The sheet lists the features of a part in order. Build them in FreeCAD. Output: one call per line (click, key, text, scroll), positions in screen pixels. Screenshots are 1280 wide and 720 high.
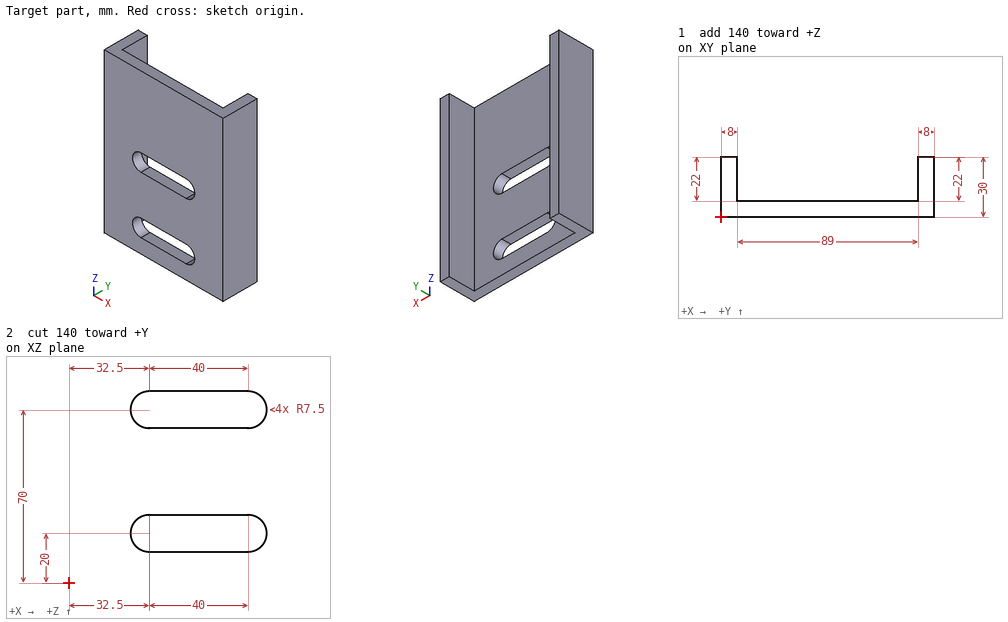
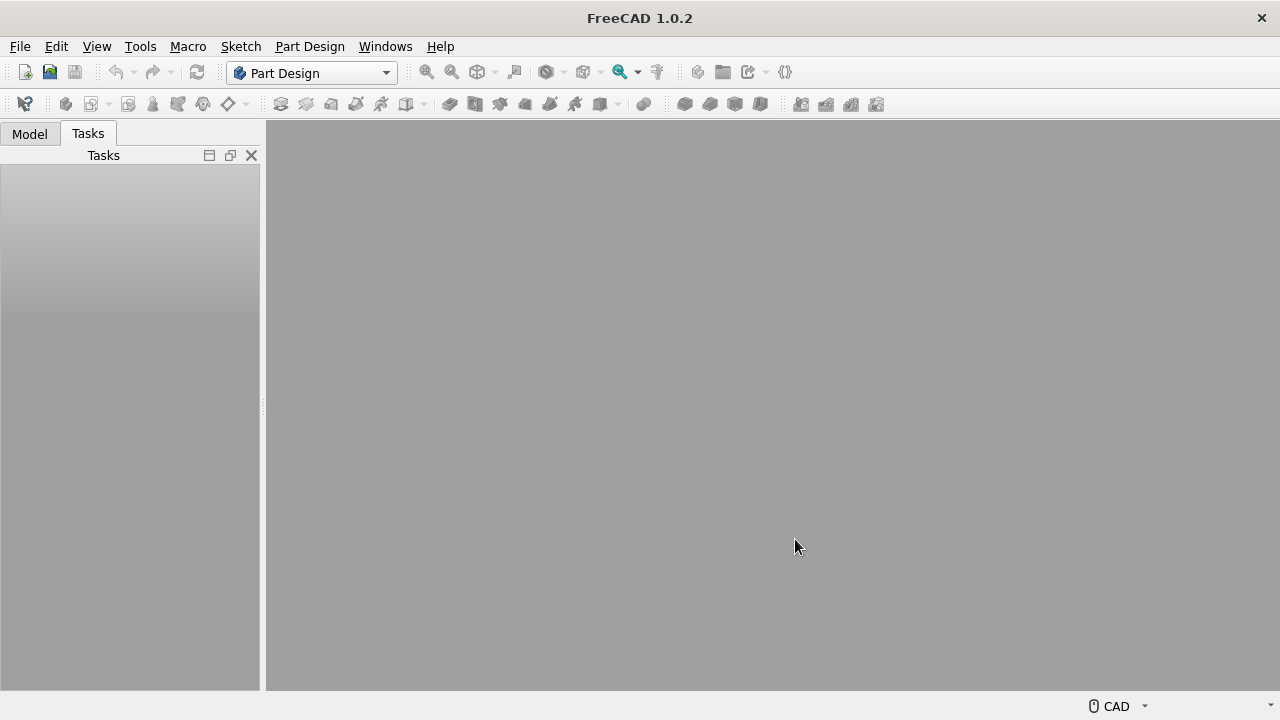
click(25, 72)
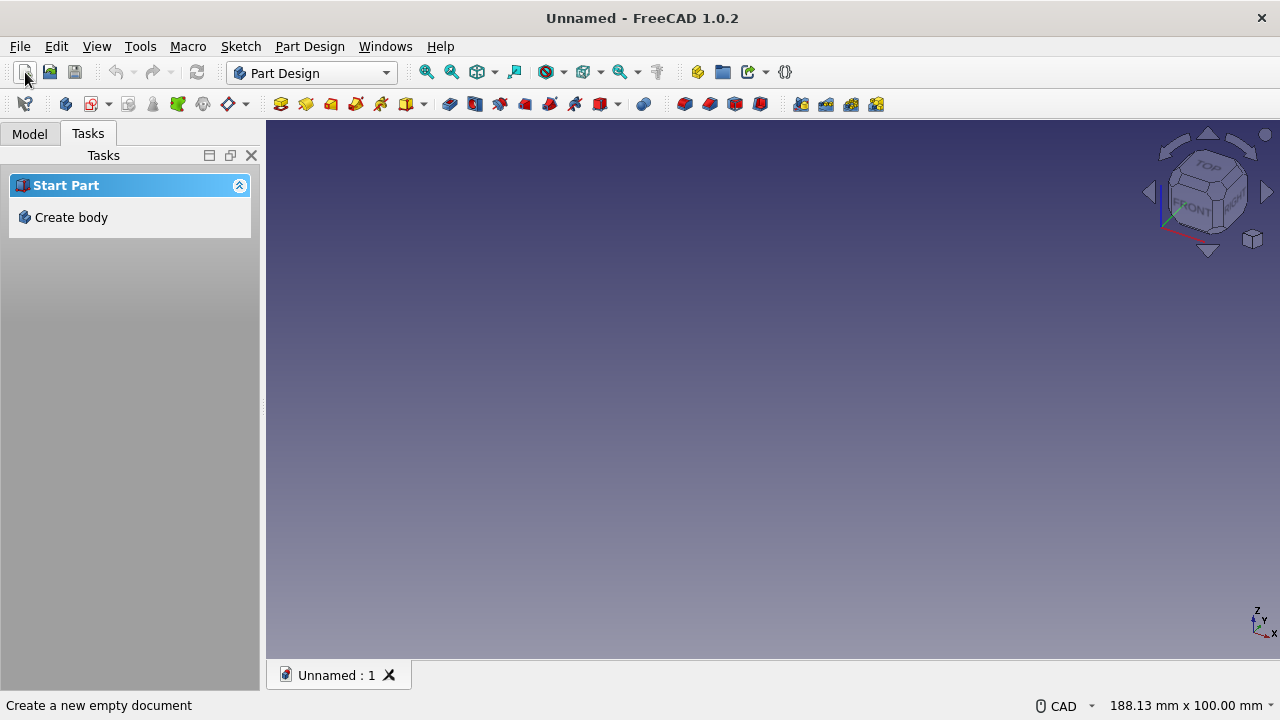
click(90, 104)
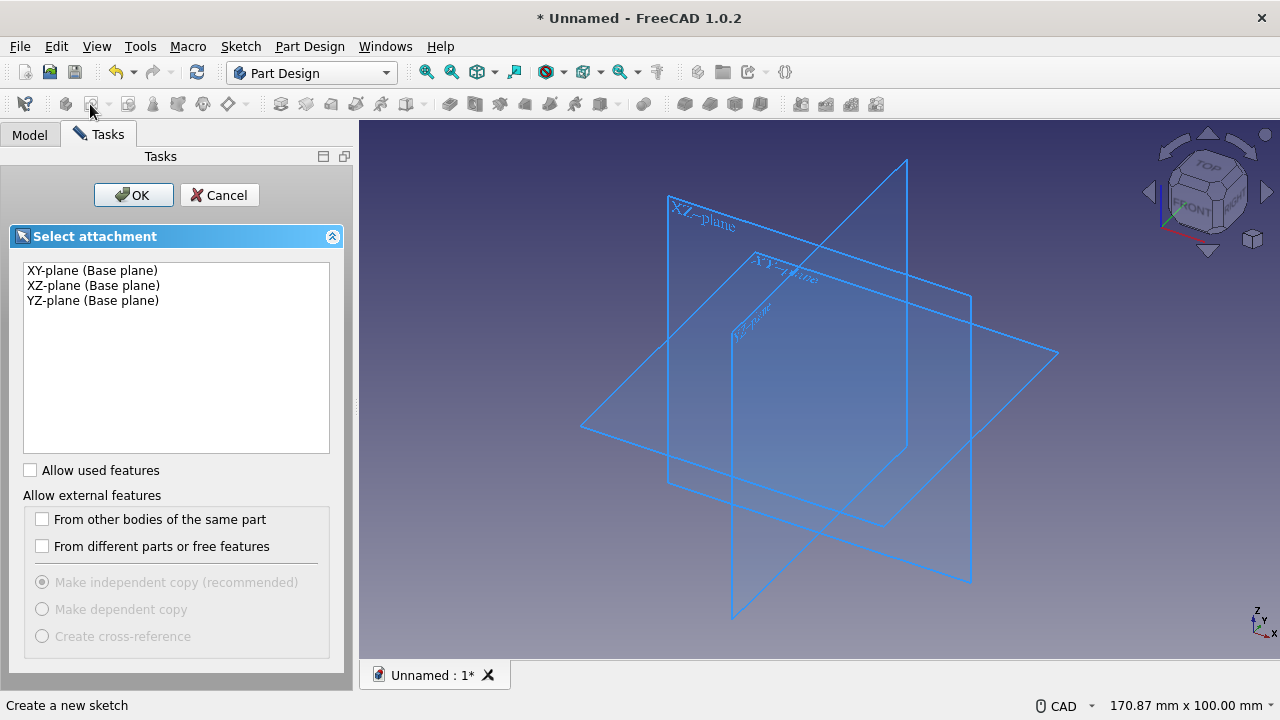
click(84, 270)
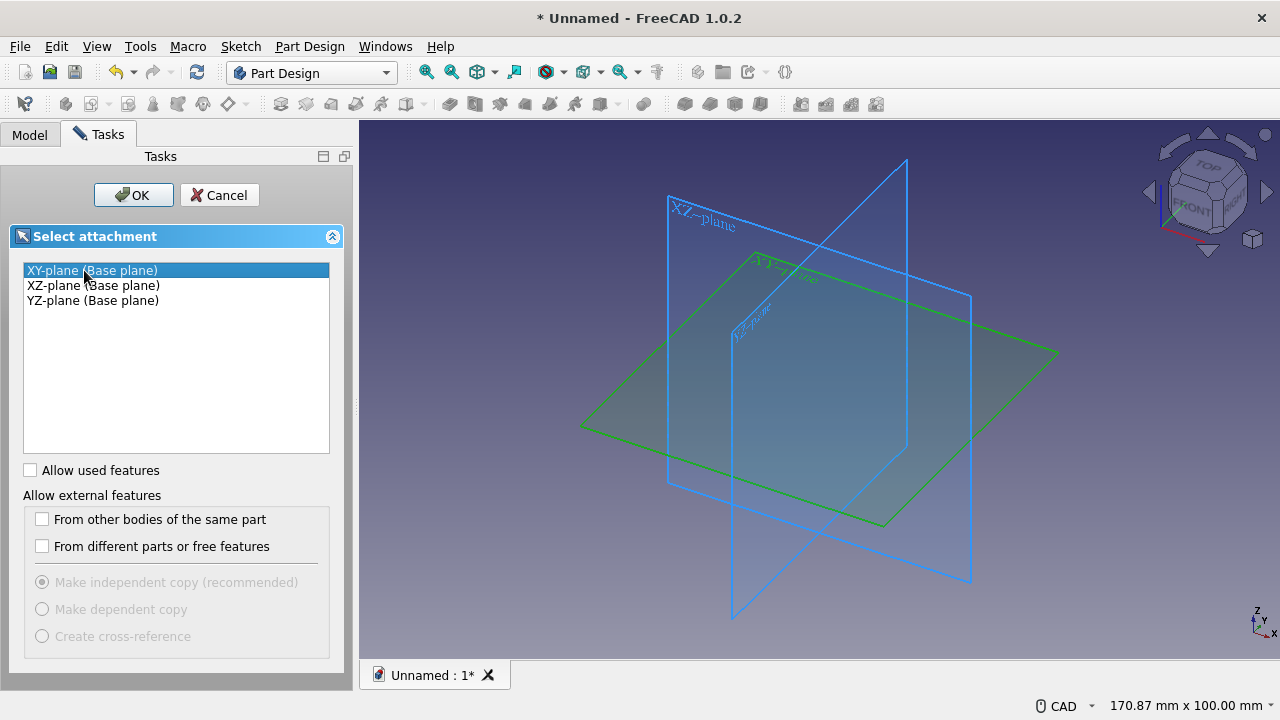
click(134, 195)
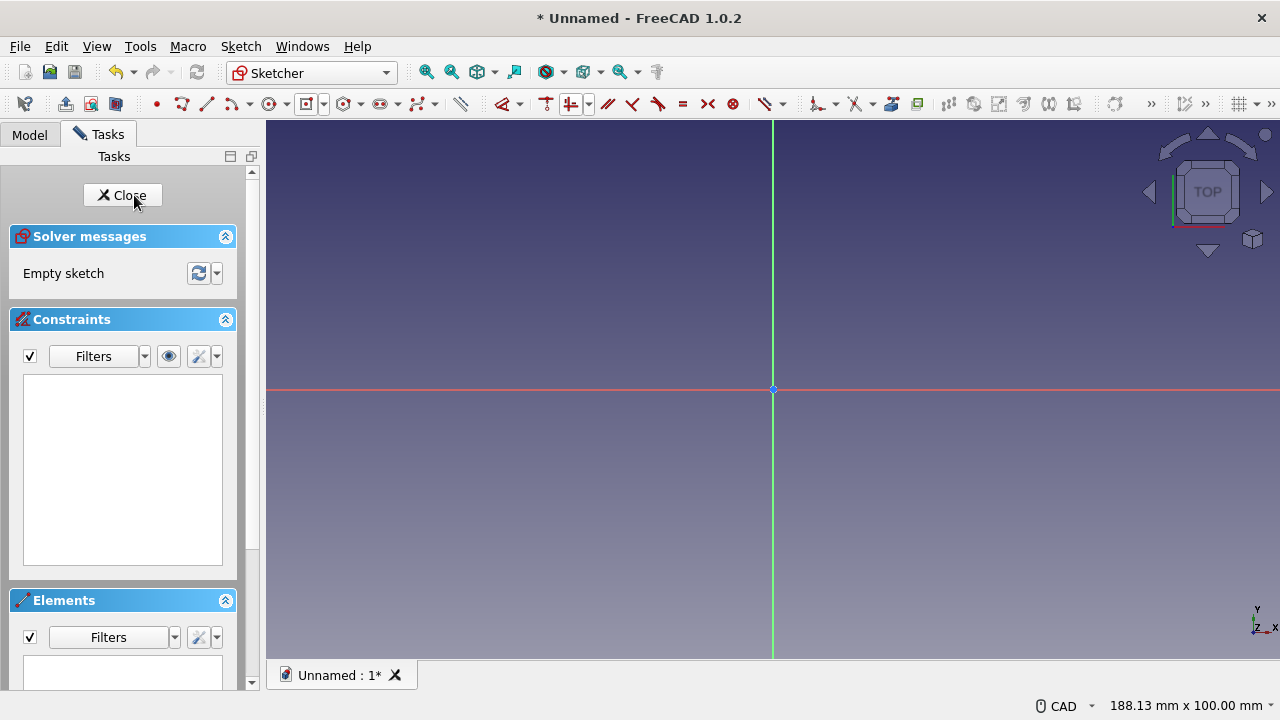
scroll(294, 554, down, 2)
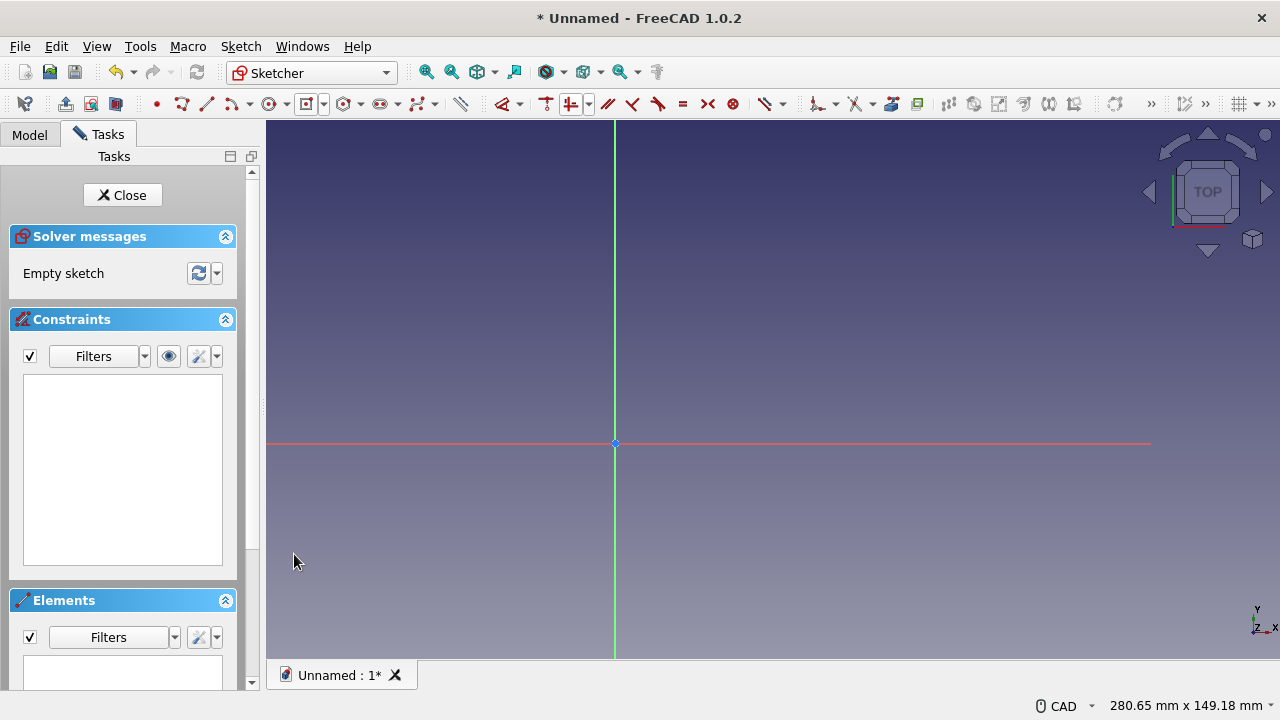
scroll(1009, 390, up, 2)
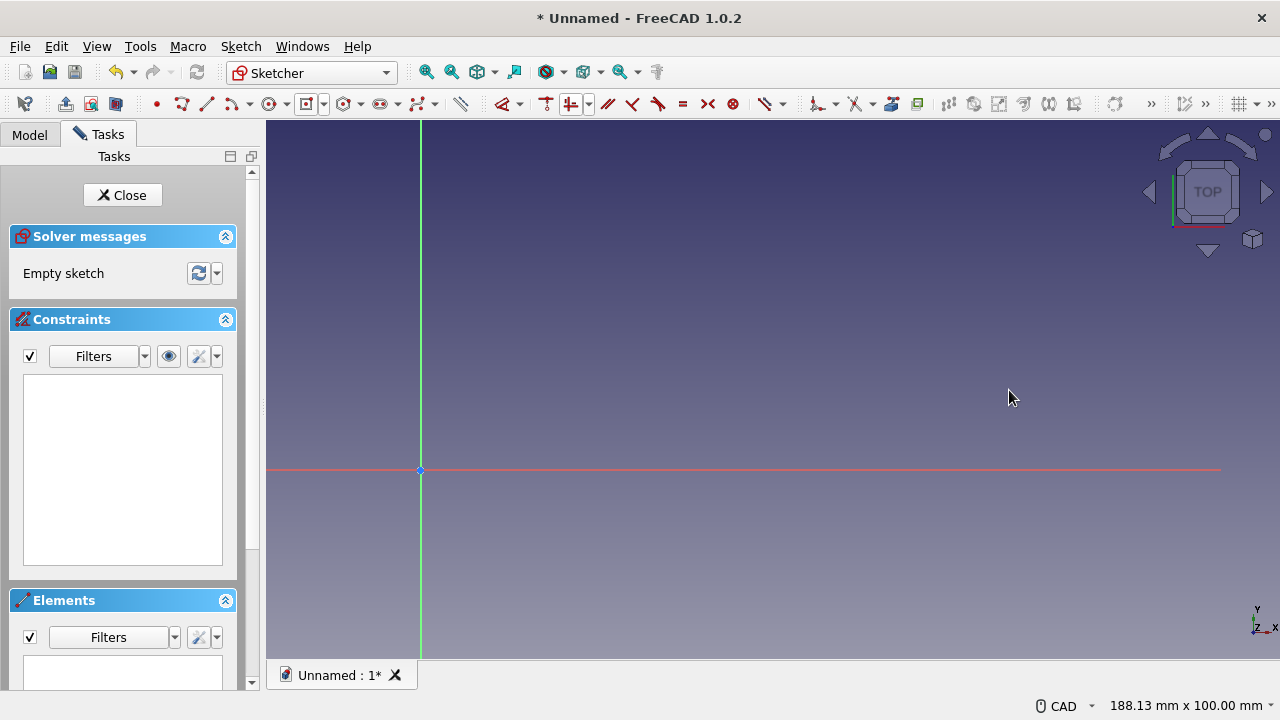
click(182, 104)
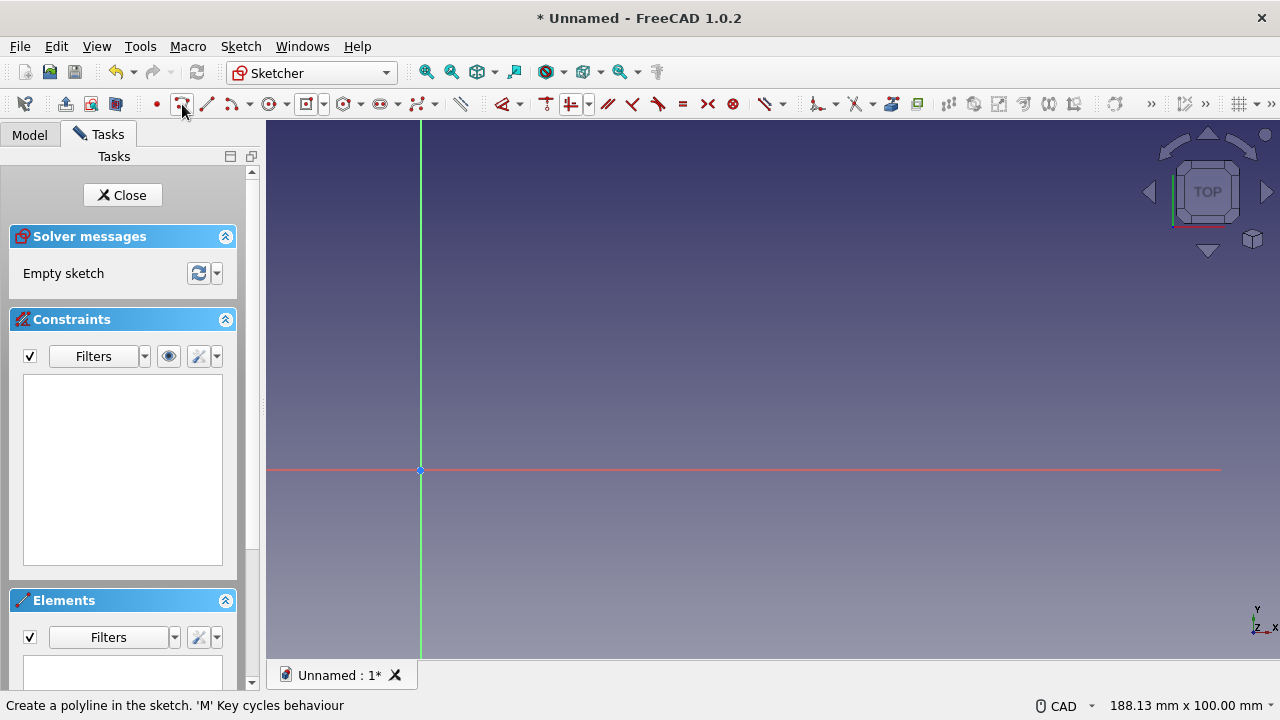
click(421, 470)
click(987, 461)
click(987, 309)
click(944, 309)
click(944, 427)
click(464, 427)
click(464, 309)
click(430, 309)
click(421, 470)
key(Escape)
key(Escape)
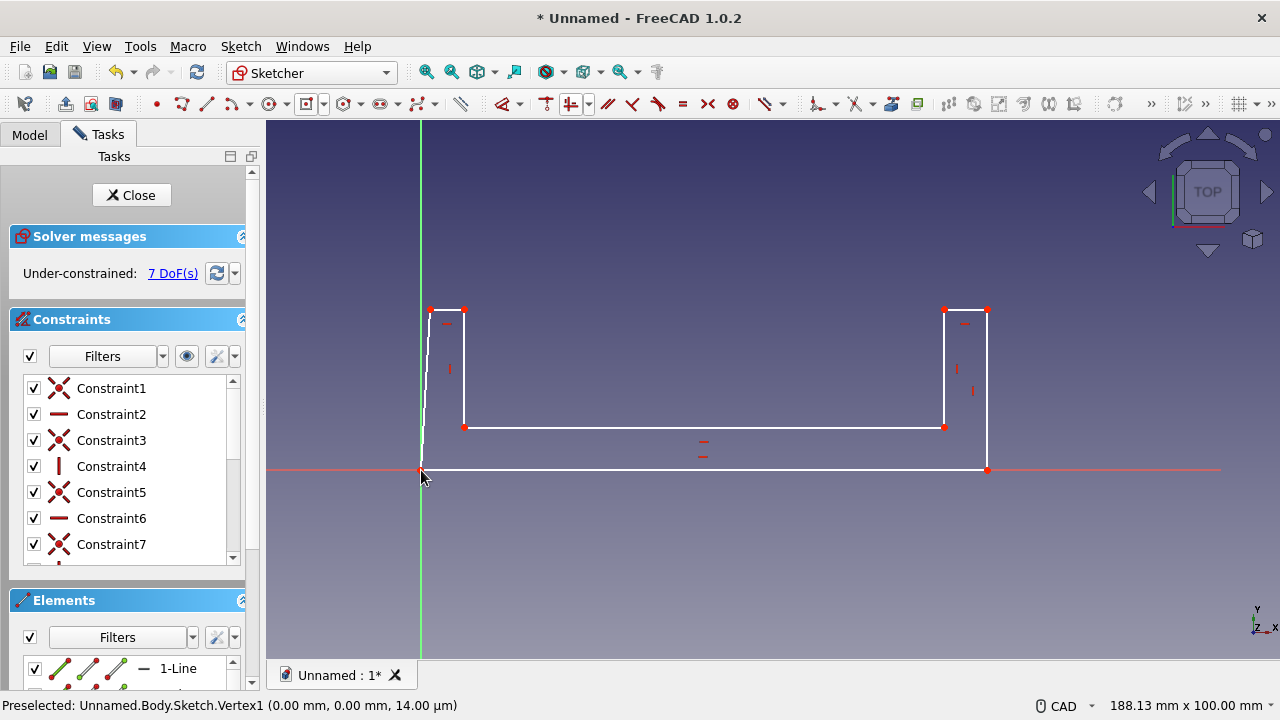
click(424, 422)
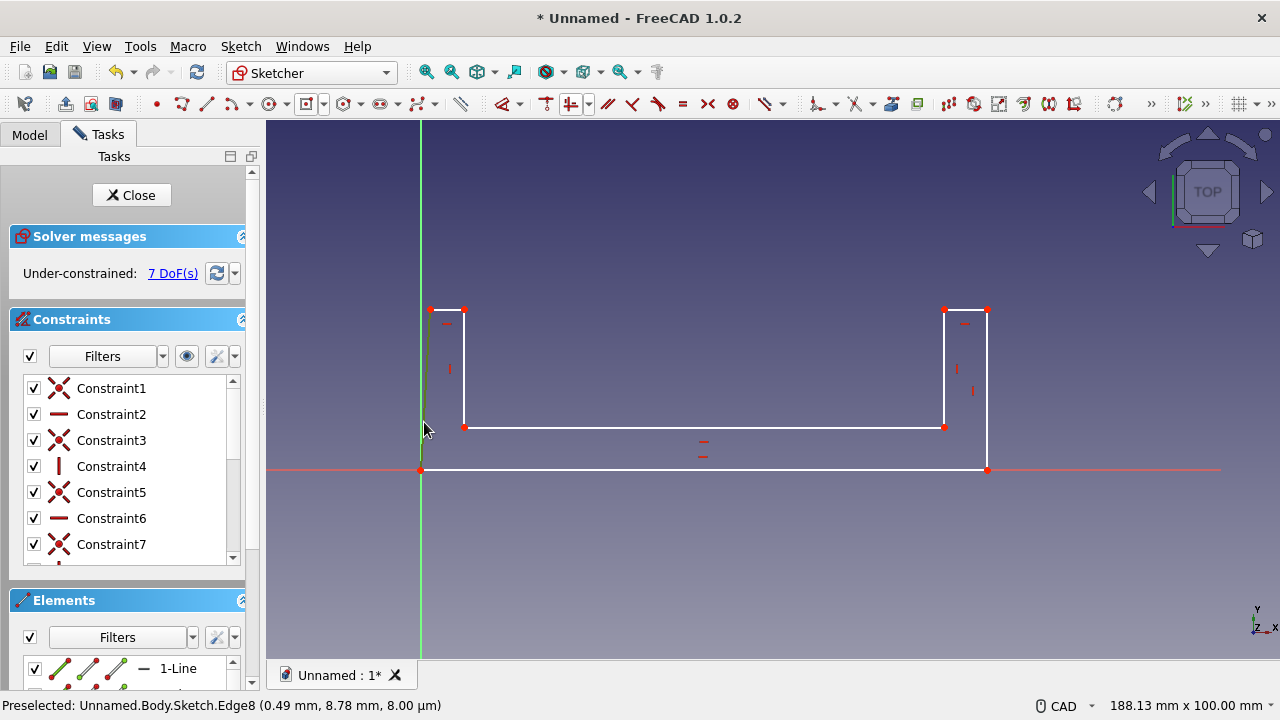
click(588, 104)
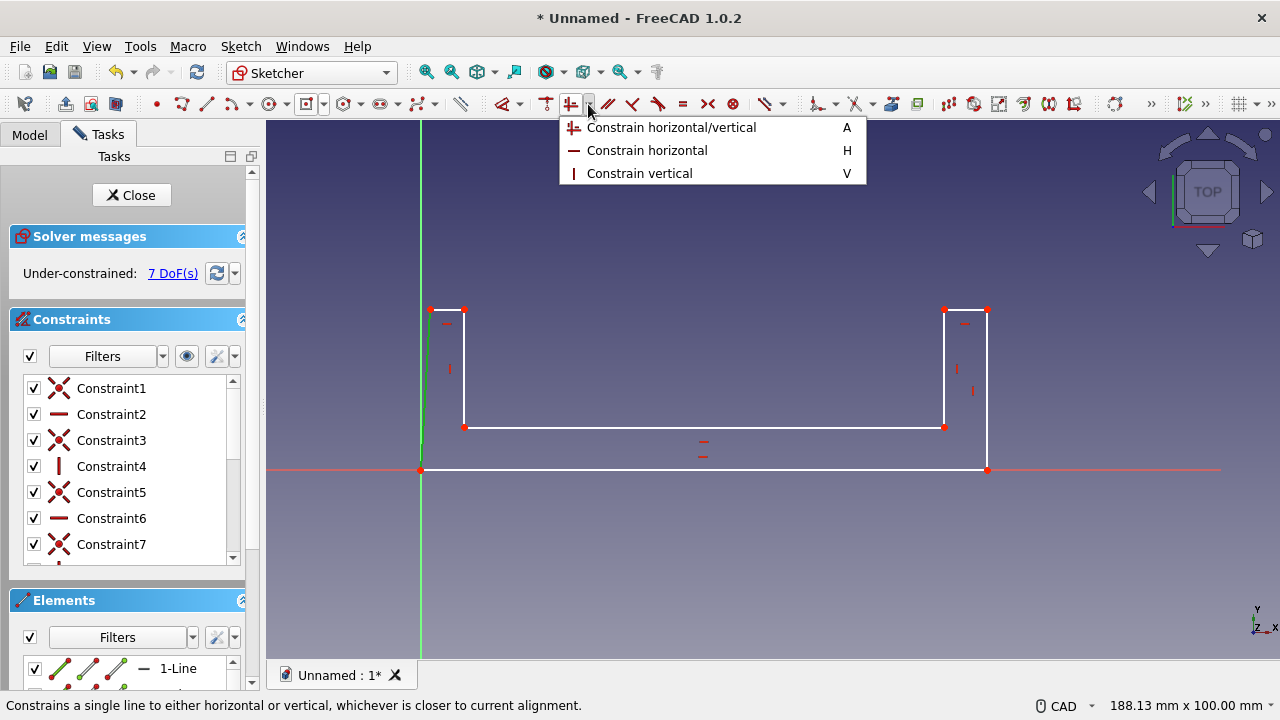
click(713, 174)